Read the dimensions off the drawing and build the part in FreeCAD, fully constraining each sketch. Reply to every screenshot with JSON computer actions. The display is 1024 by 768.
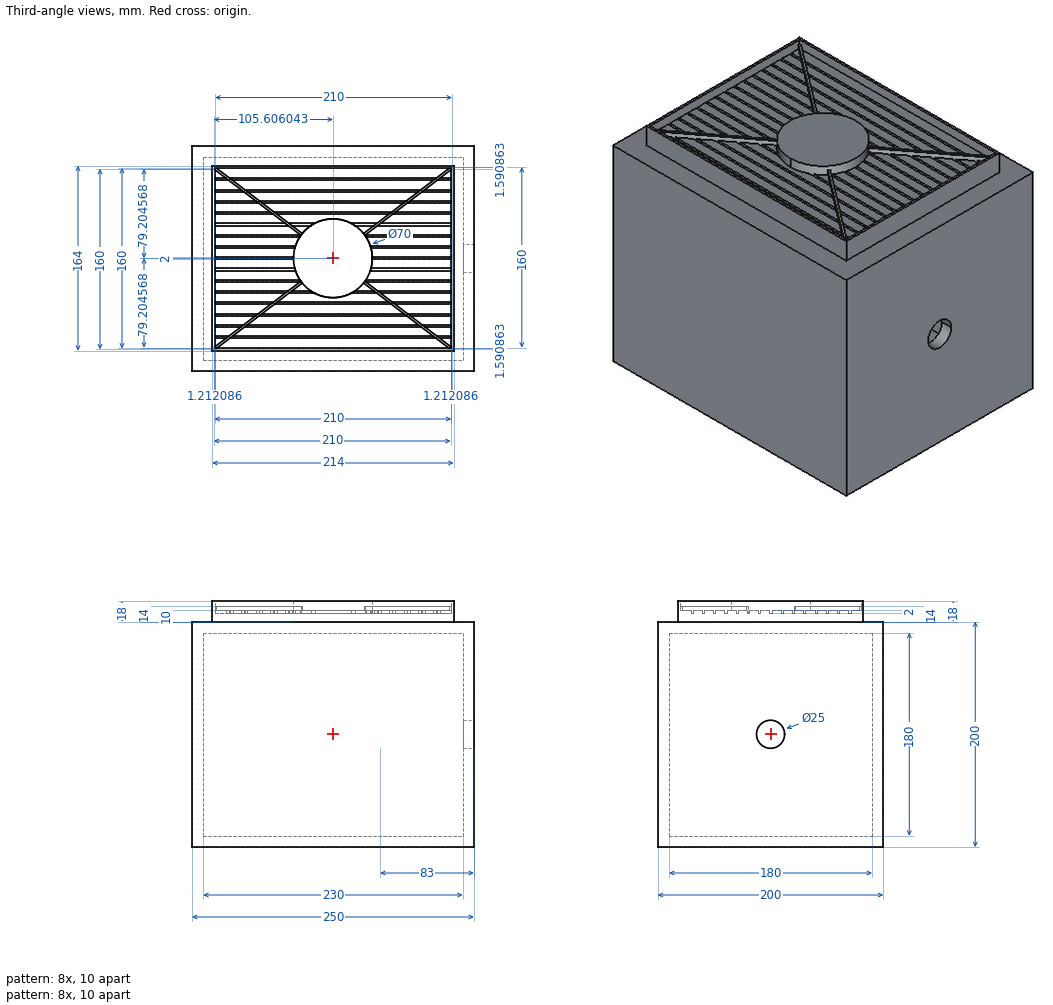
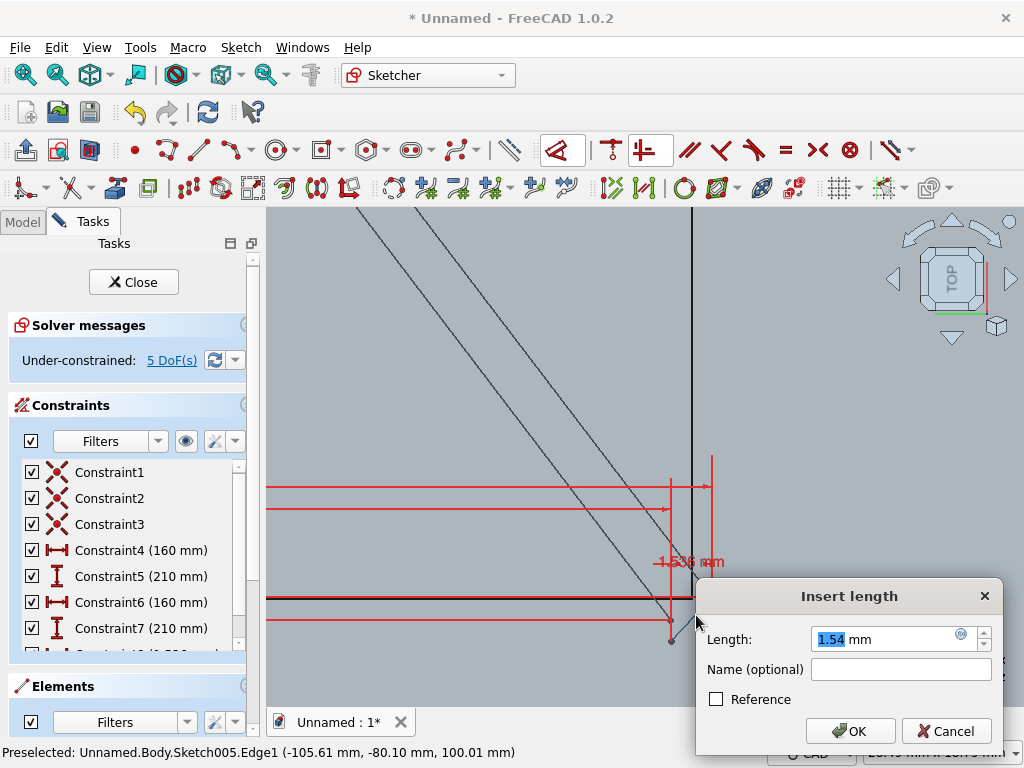
{"action": "type", "text": "1.590863"}
{"action": "key", "text": "Return"}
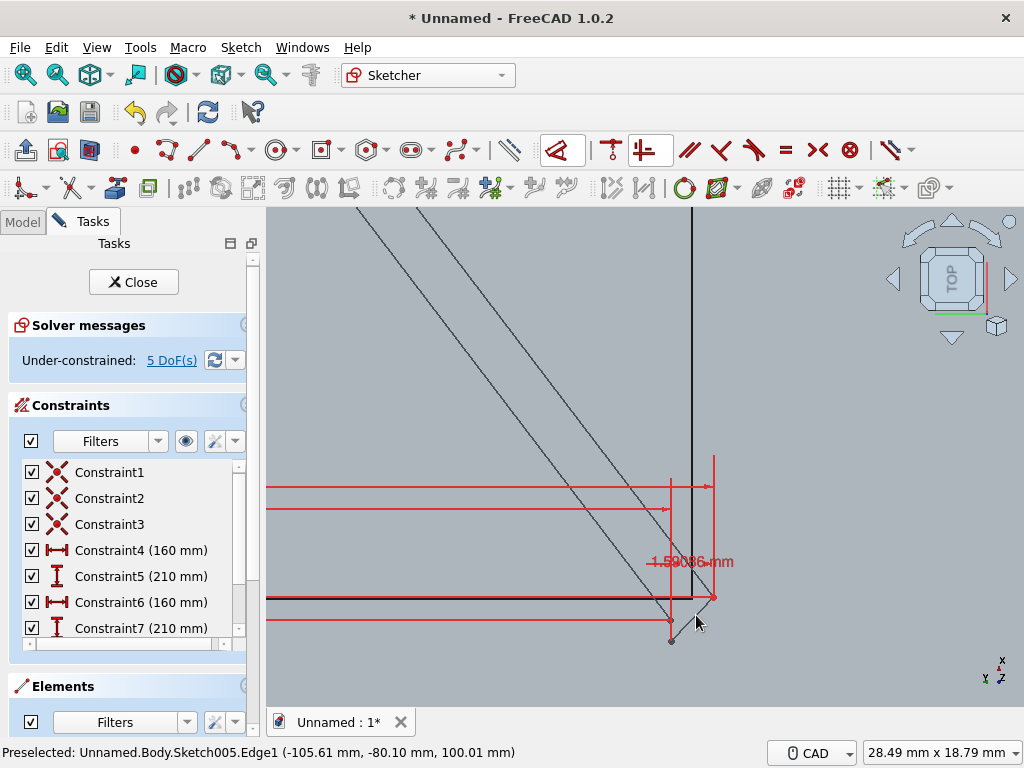
{"action": "scroll", "coordinate": [684, 628], "scroll_direction": "up", "scroll_amount": 2}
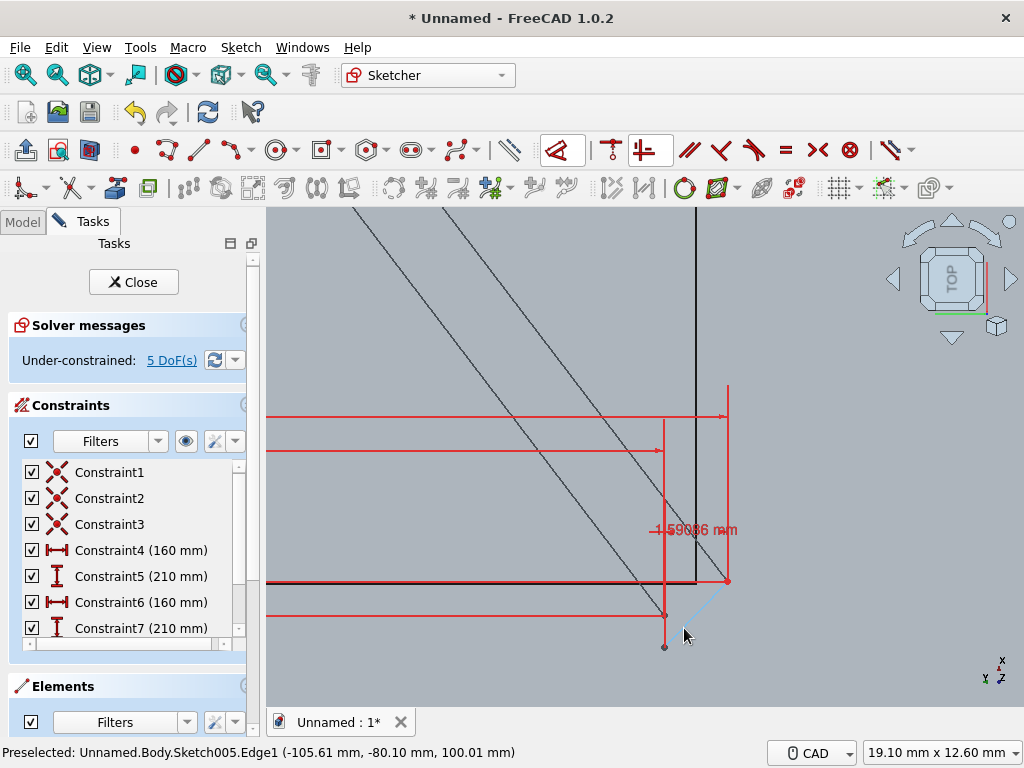
{"action": "left_click", "coordinate": [684, 628]}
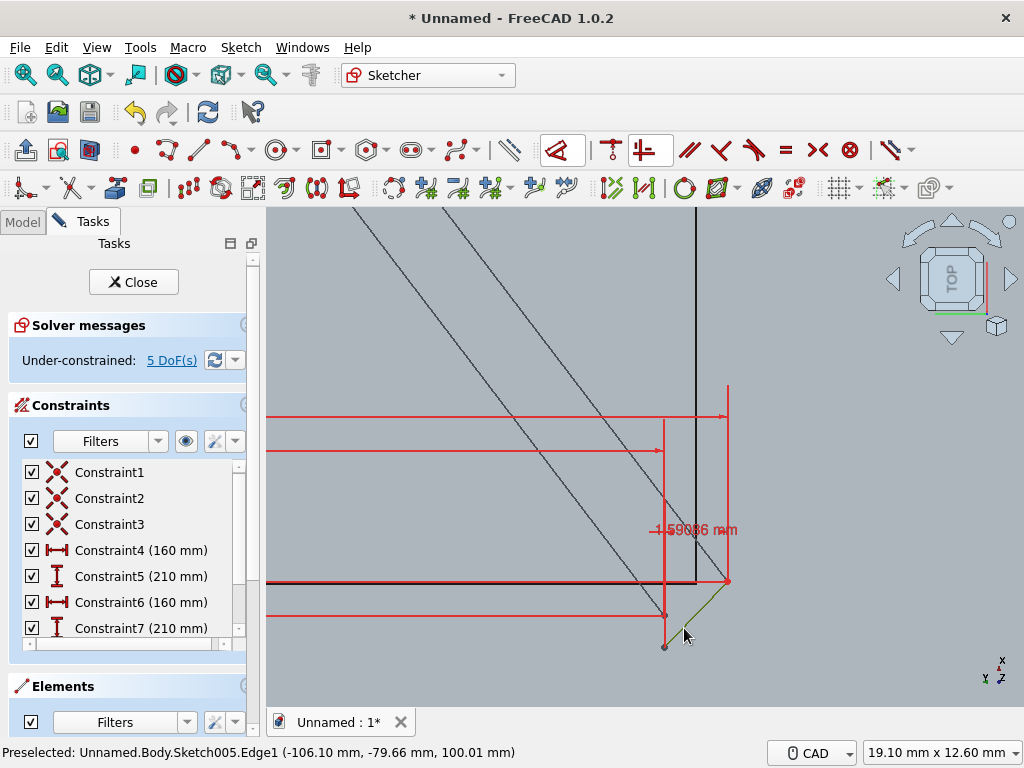
{"action": "key", "text": "i"}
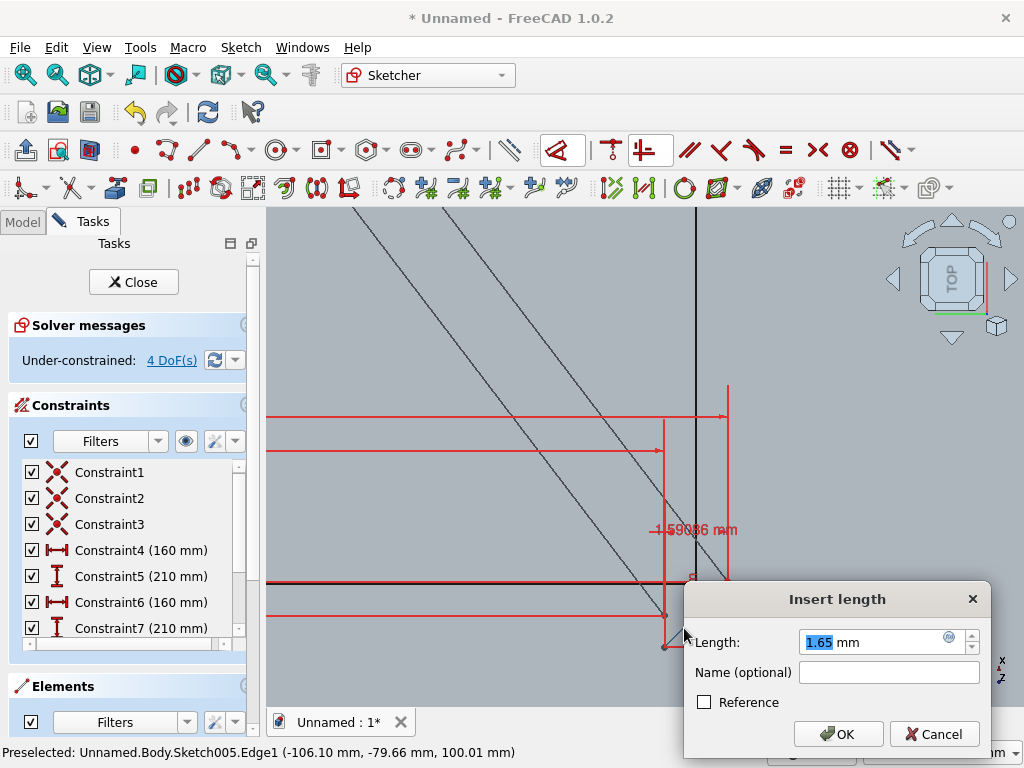
{"action": "type", "text": "1.212086"}
{"action": "key", "text": "Return"}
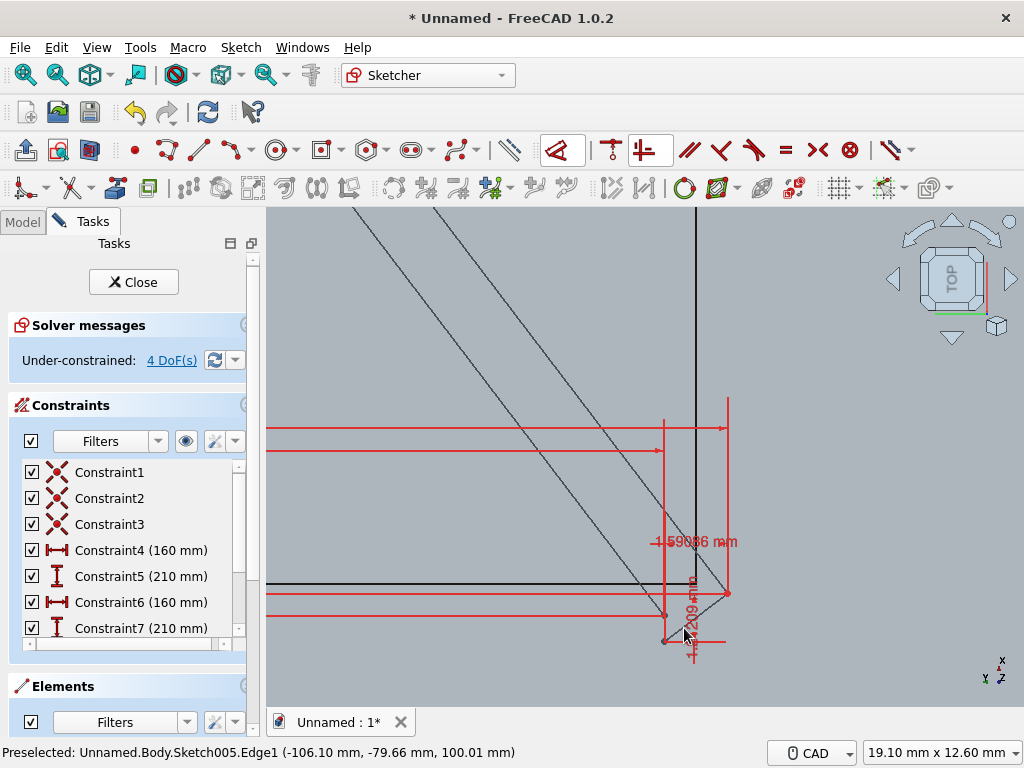
{"action": "scroll", "coordinate": [706, 629], "scroll_direction": "down", "scroll_amount": 16}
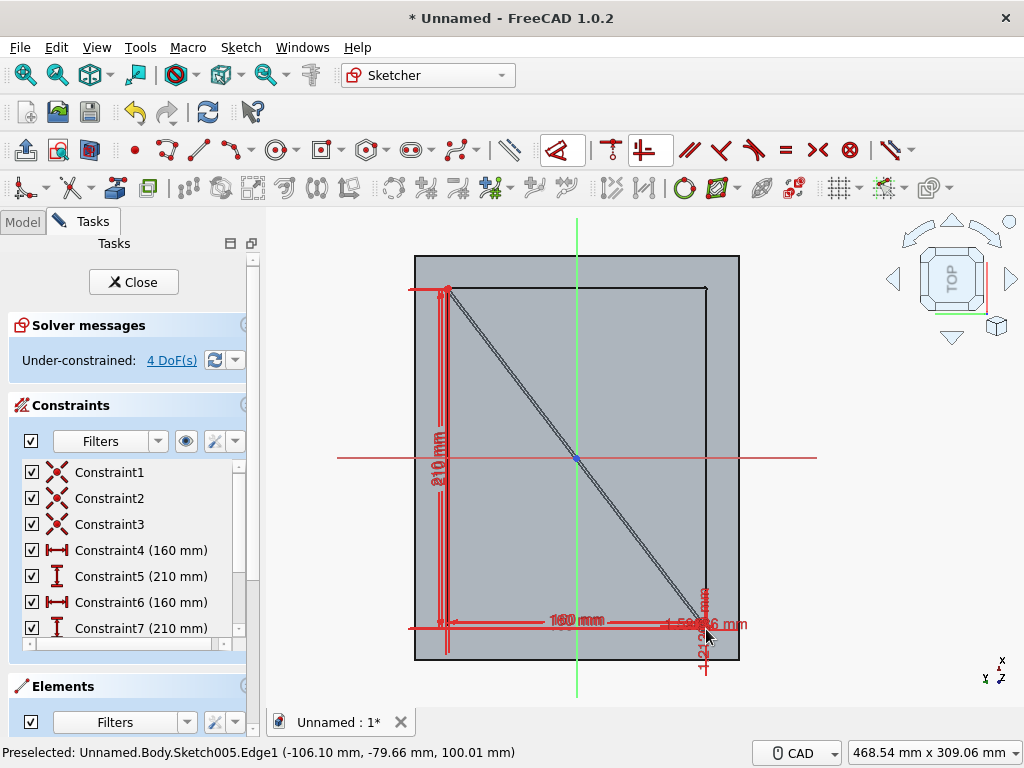
{"action": "scroll", "coordinate": [448, 289], "scroll_direction": "up", "scroll_amount": 14}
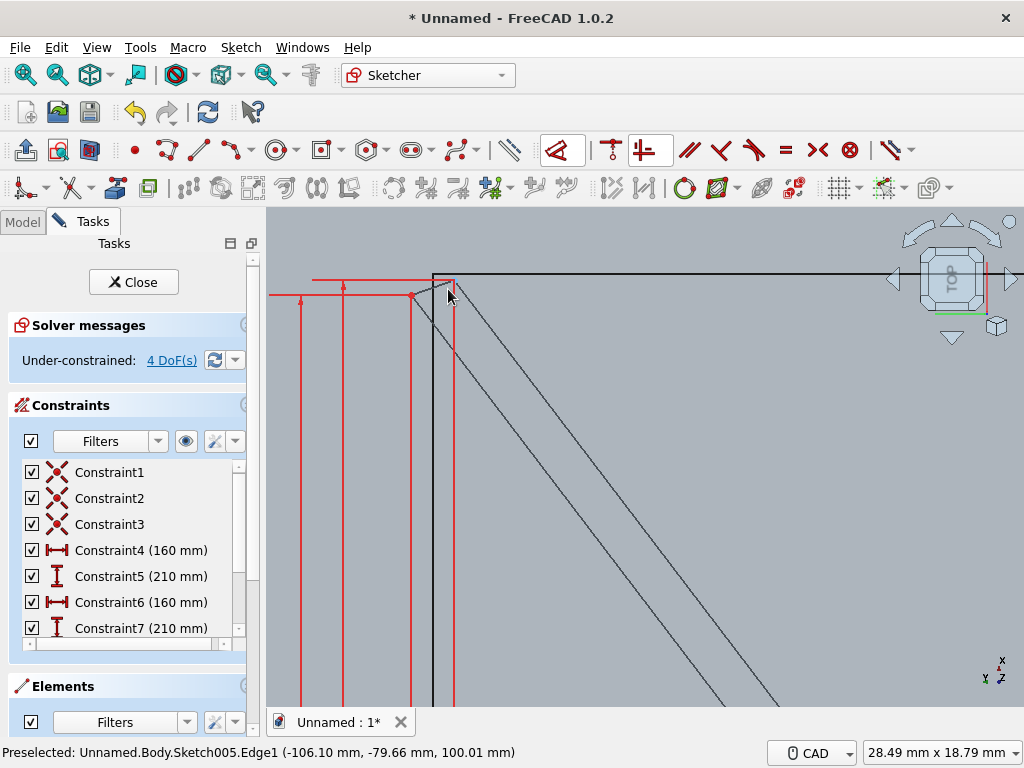
{"action": "left_click", "coordinate": [441, 285]}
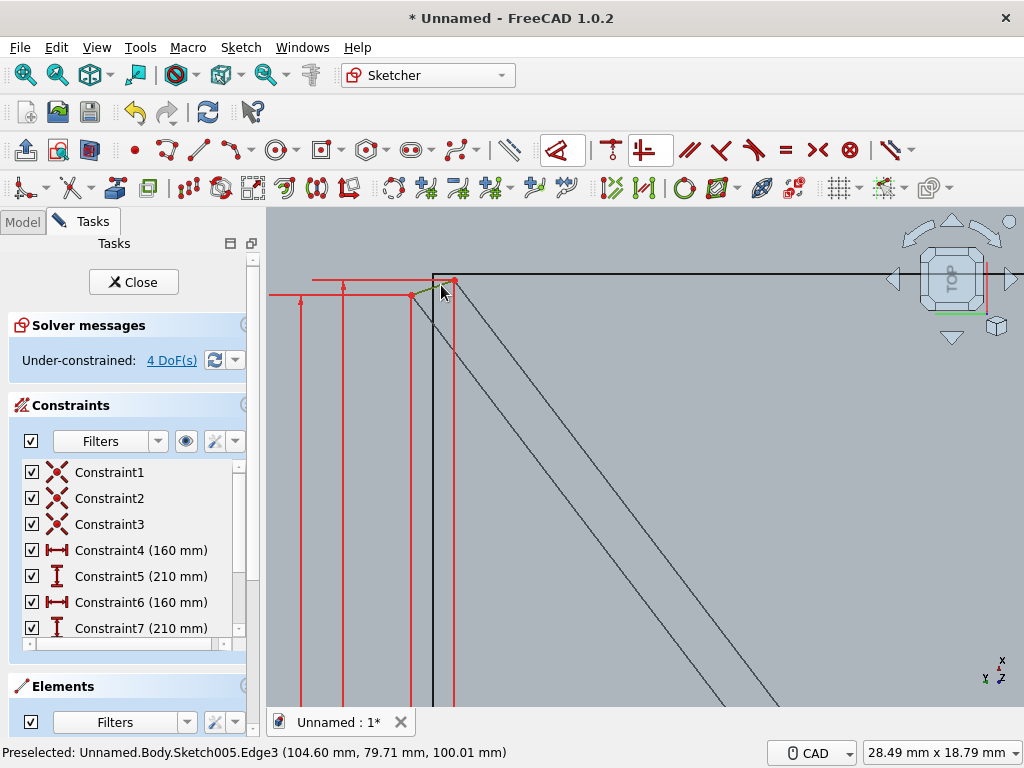
{"action": "left_click", "coordinate": [580, 150]}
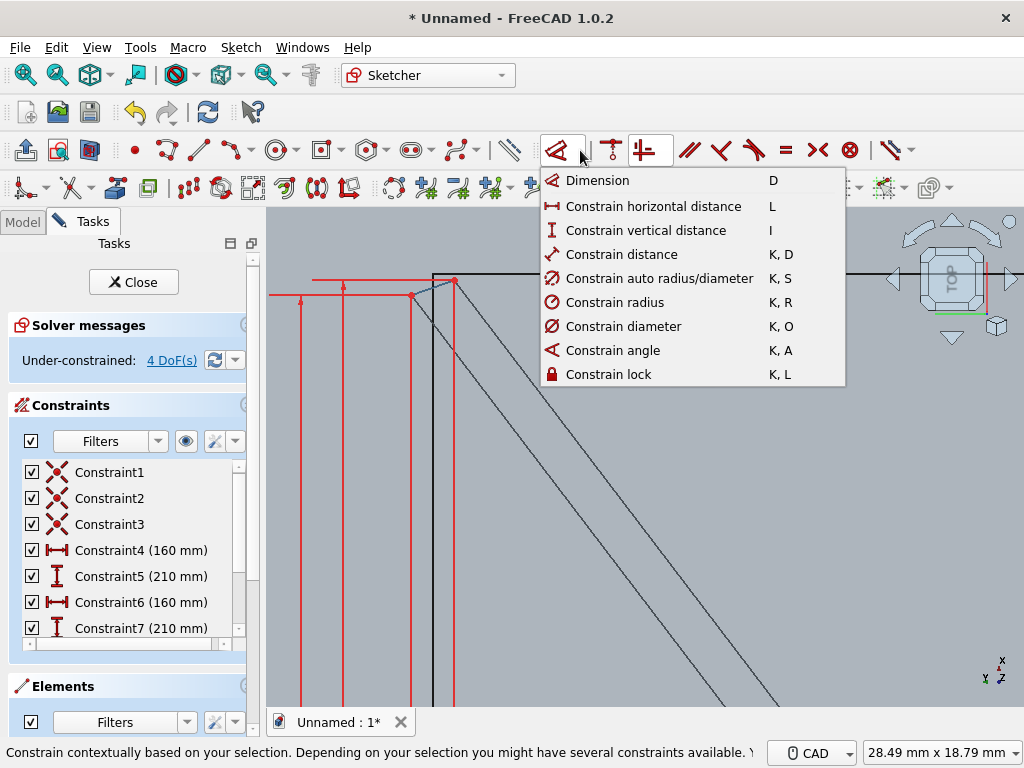
{"action": "left_click", "coordinate": [693, 206]}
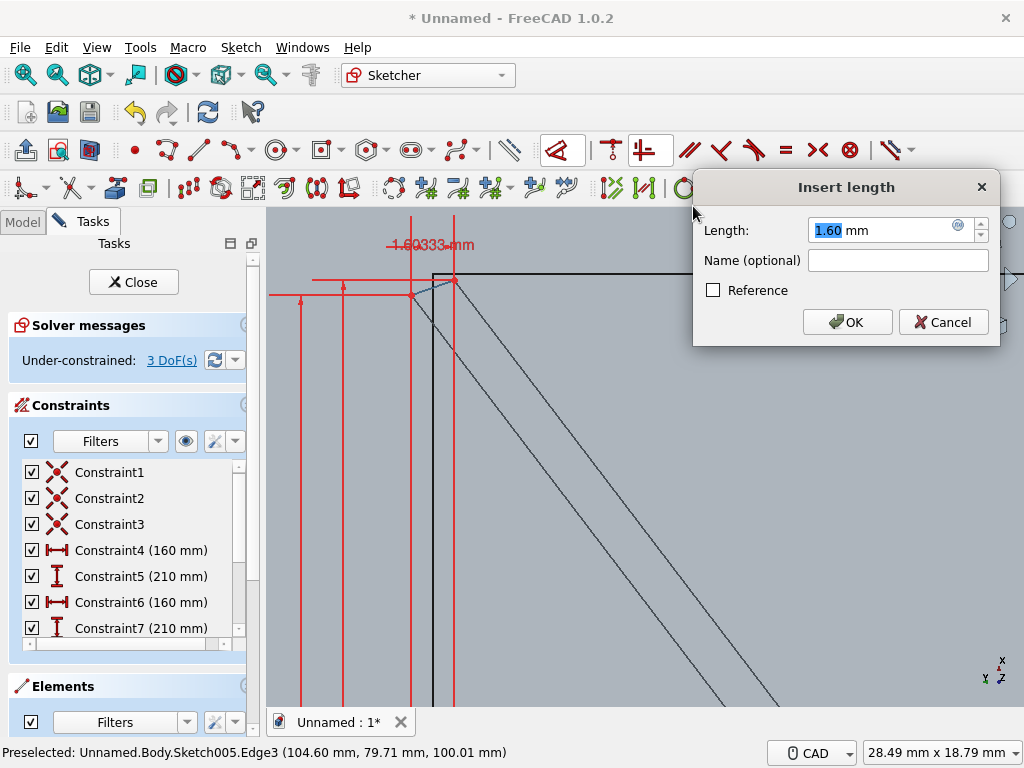
{"action": "type", "text": "1.590863"}
{"action": "key", "text": "Return"}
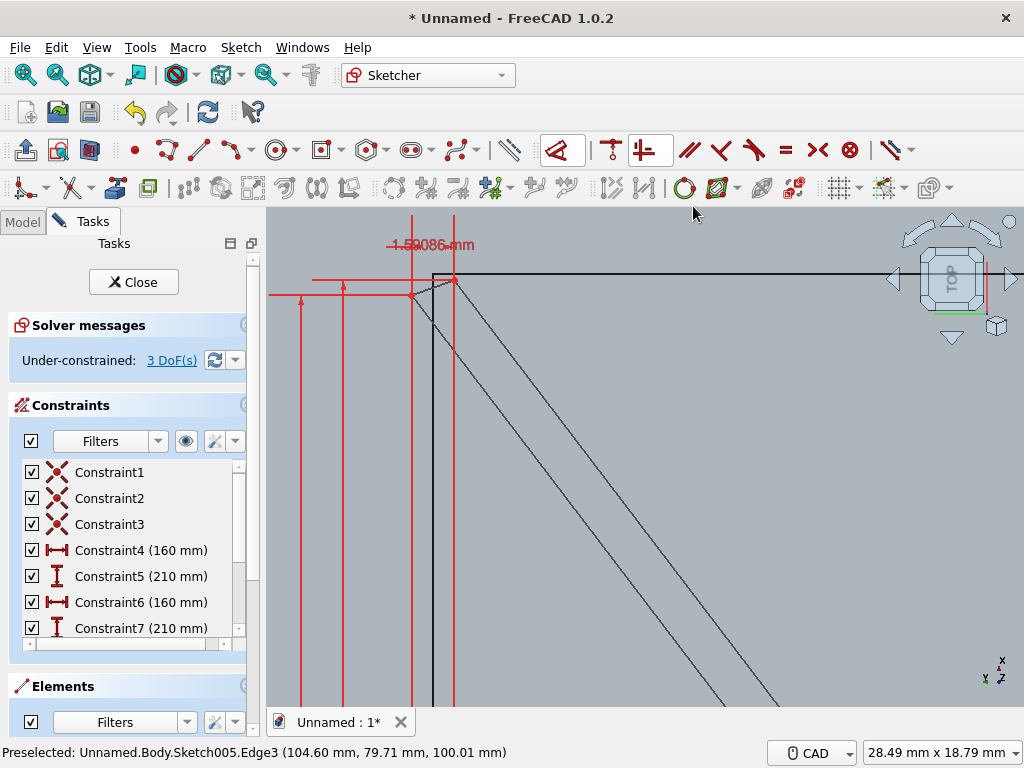
{"action": "scroll", "coordinate": [441, 285], "scroll_direction": "up", "scroll_amount": 2}